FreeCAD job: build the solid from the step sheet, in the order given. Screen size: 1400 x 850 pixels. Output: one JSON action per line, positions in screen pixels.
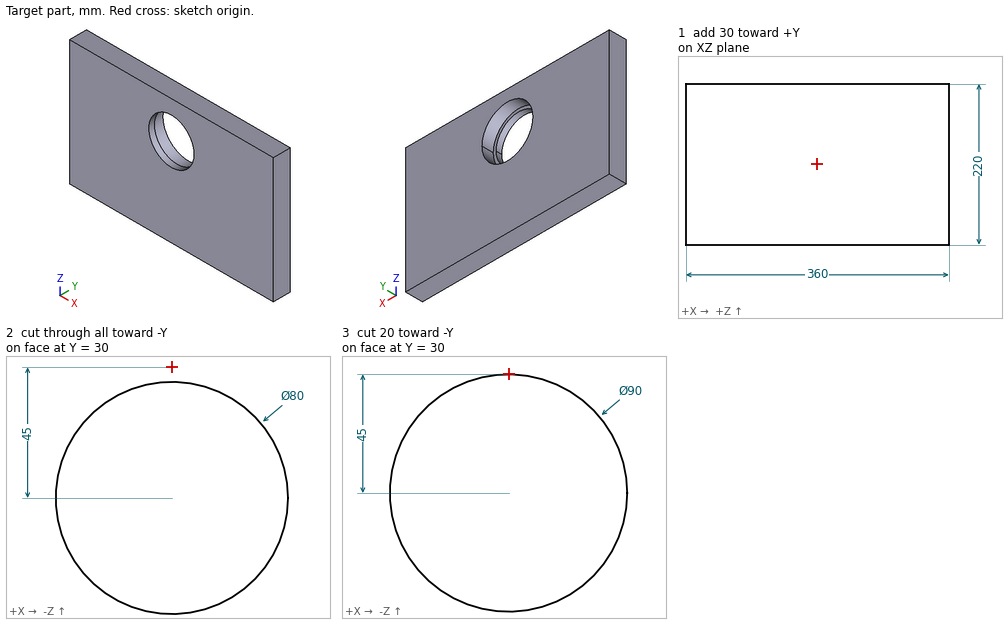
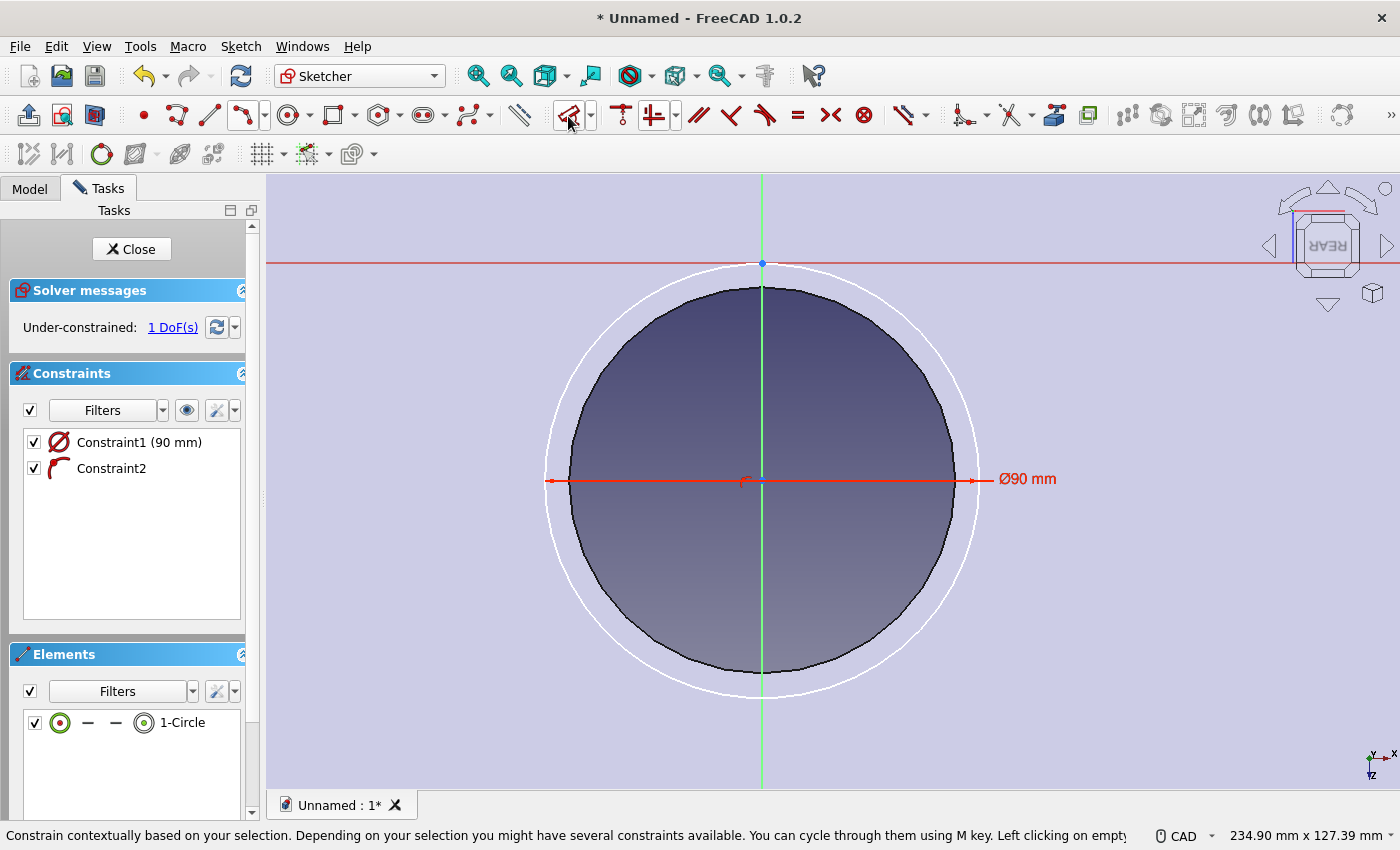
{"action": "left_click", "coordinate": [762, 481]}
{"action": "left_click", "coordinate": [796, 372]}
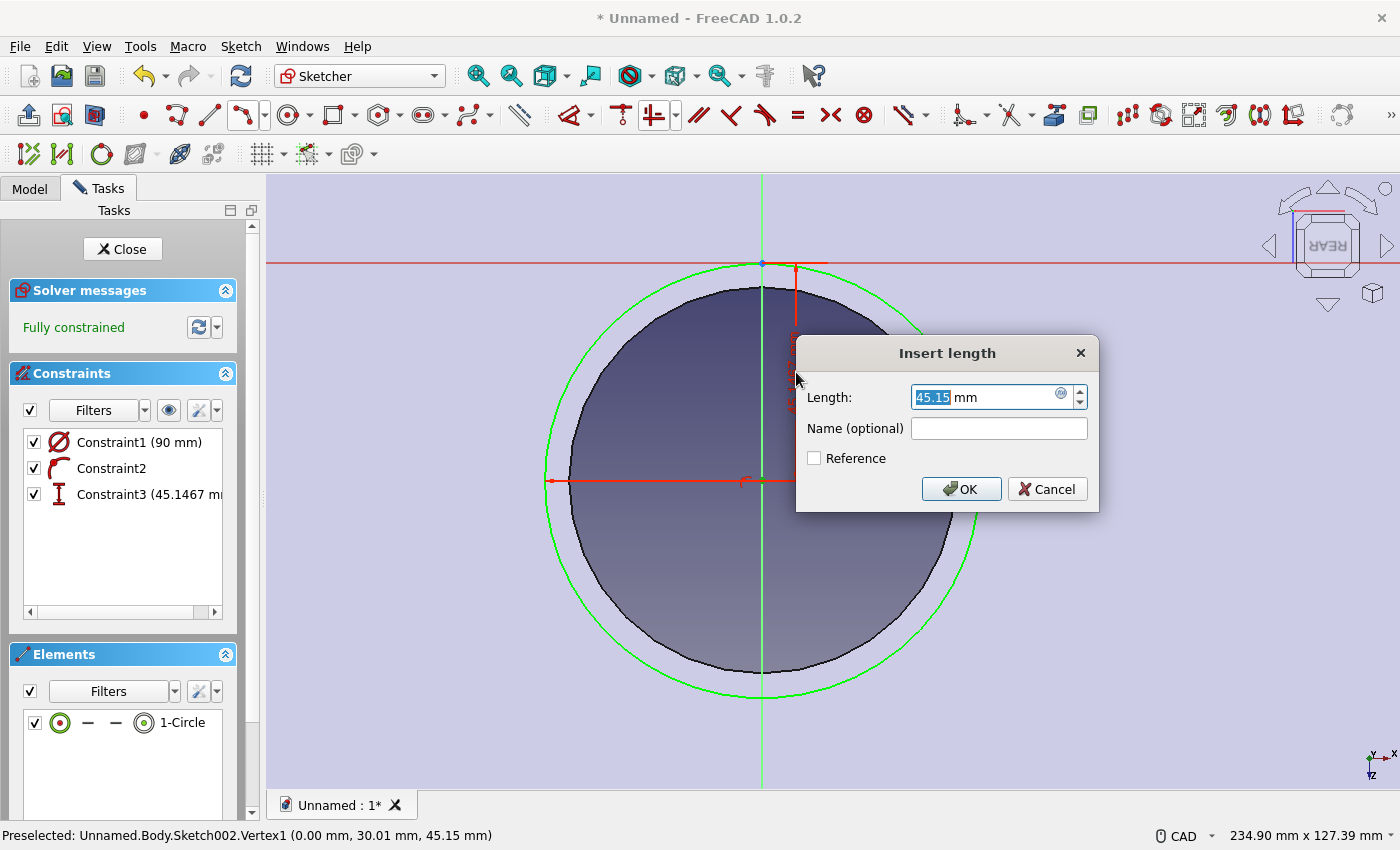
{"action": "type", "text": "45"}
{"action": "key", "text": "Return"}
{"action": "key", "text": "Escape"}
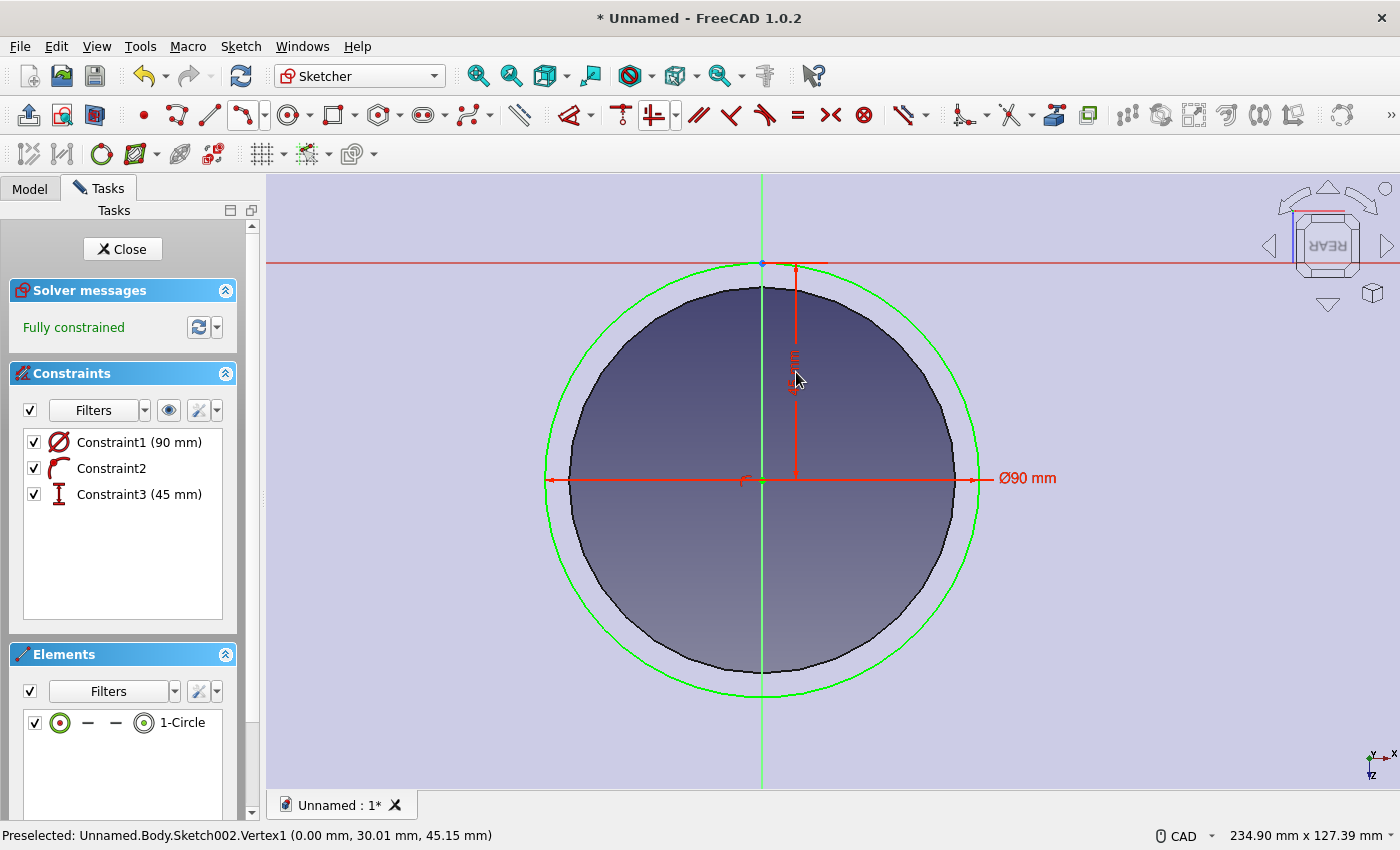
{"action": "left_click", "coordinate": [123, 249]}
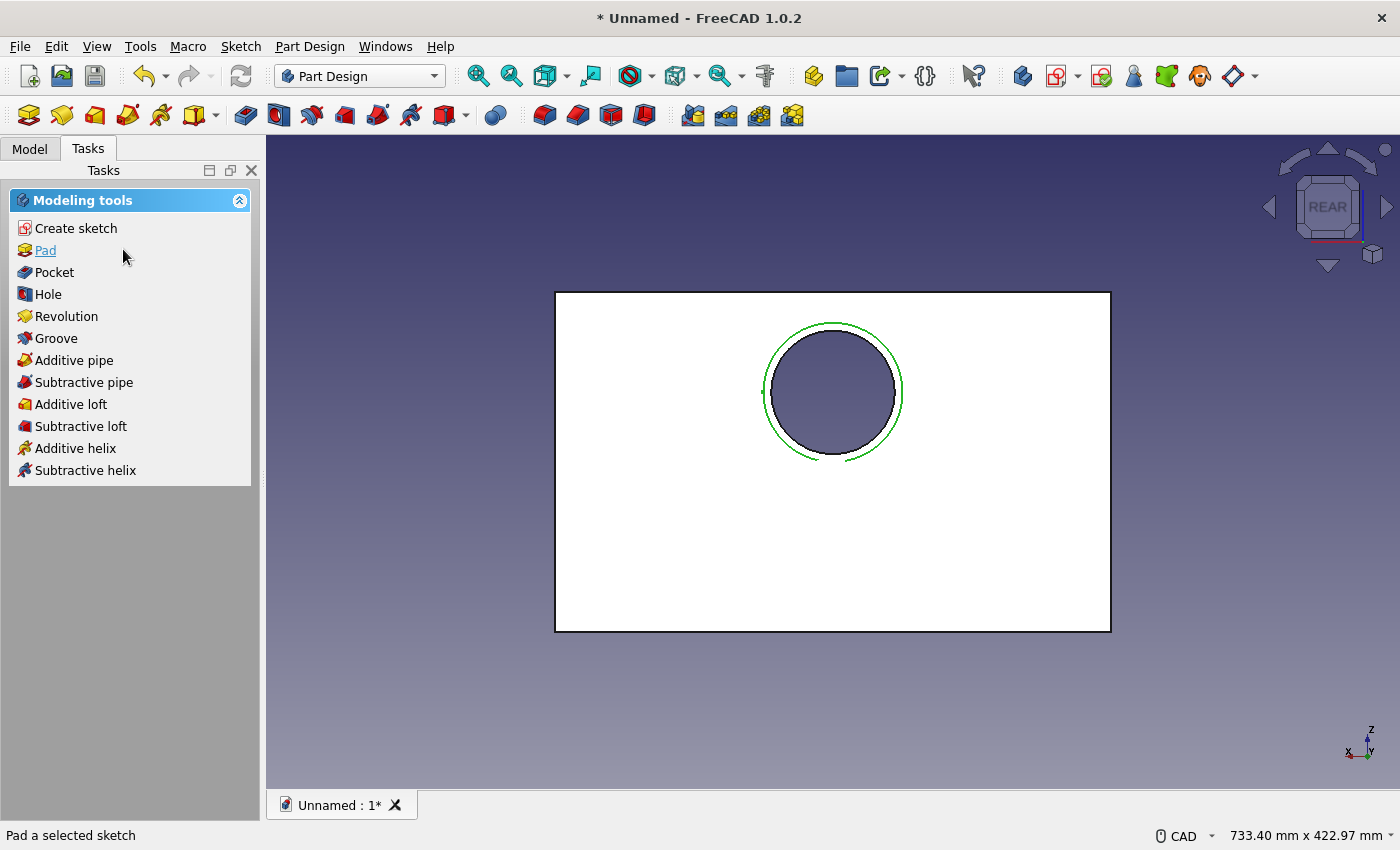
{"action": "left_click", "coordinate": [246, 116]}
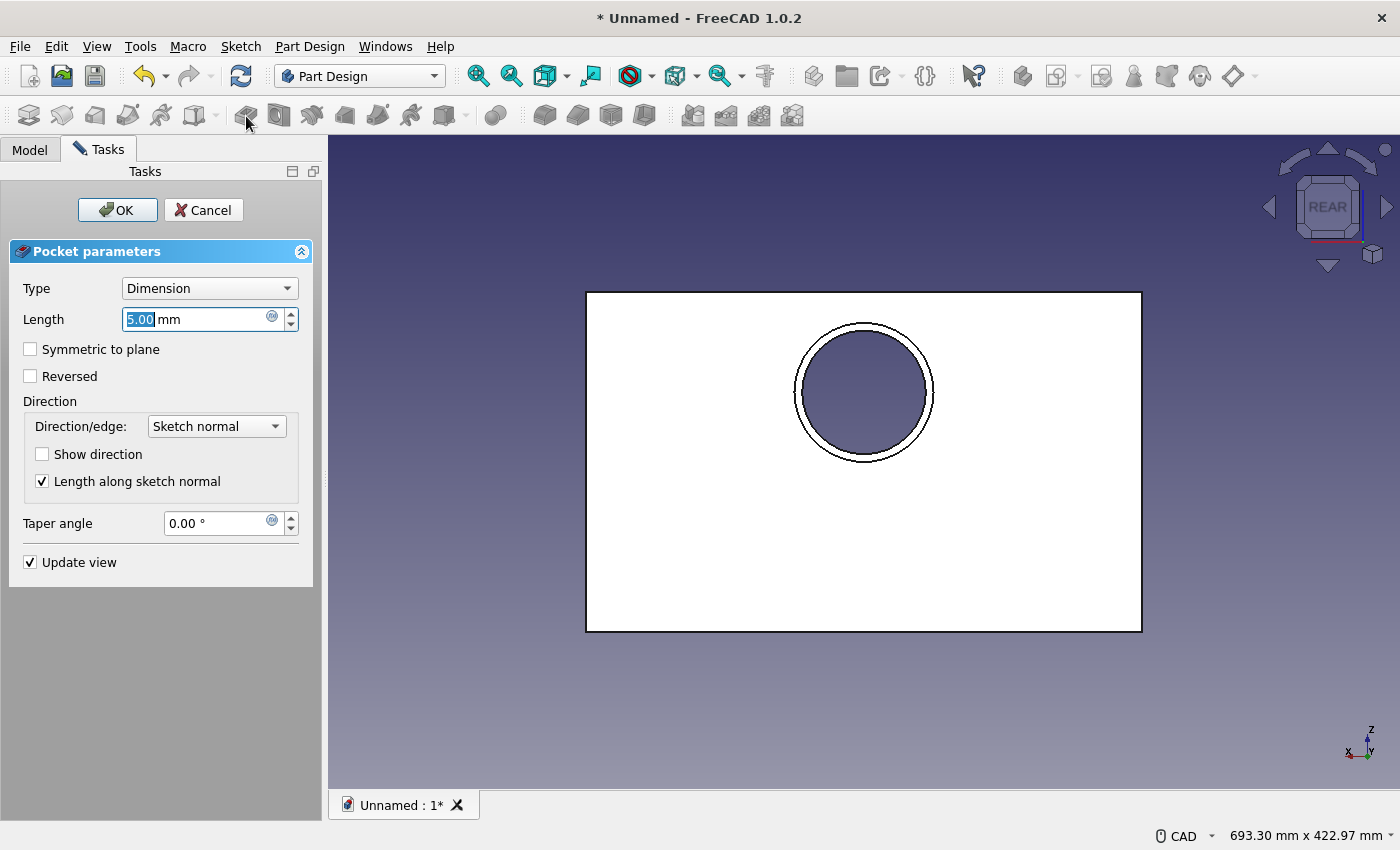
{"action": "type", "text": "20"}
{"action": "key", "text": "Tab"}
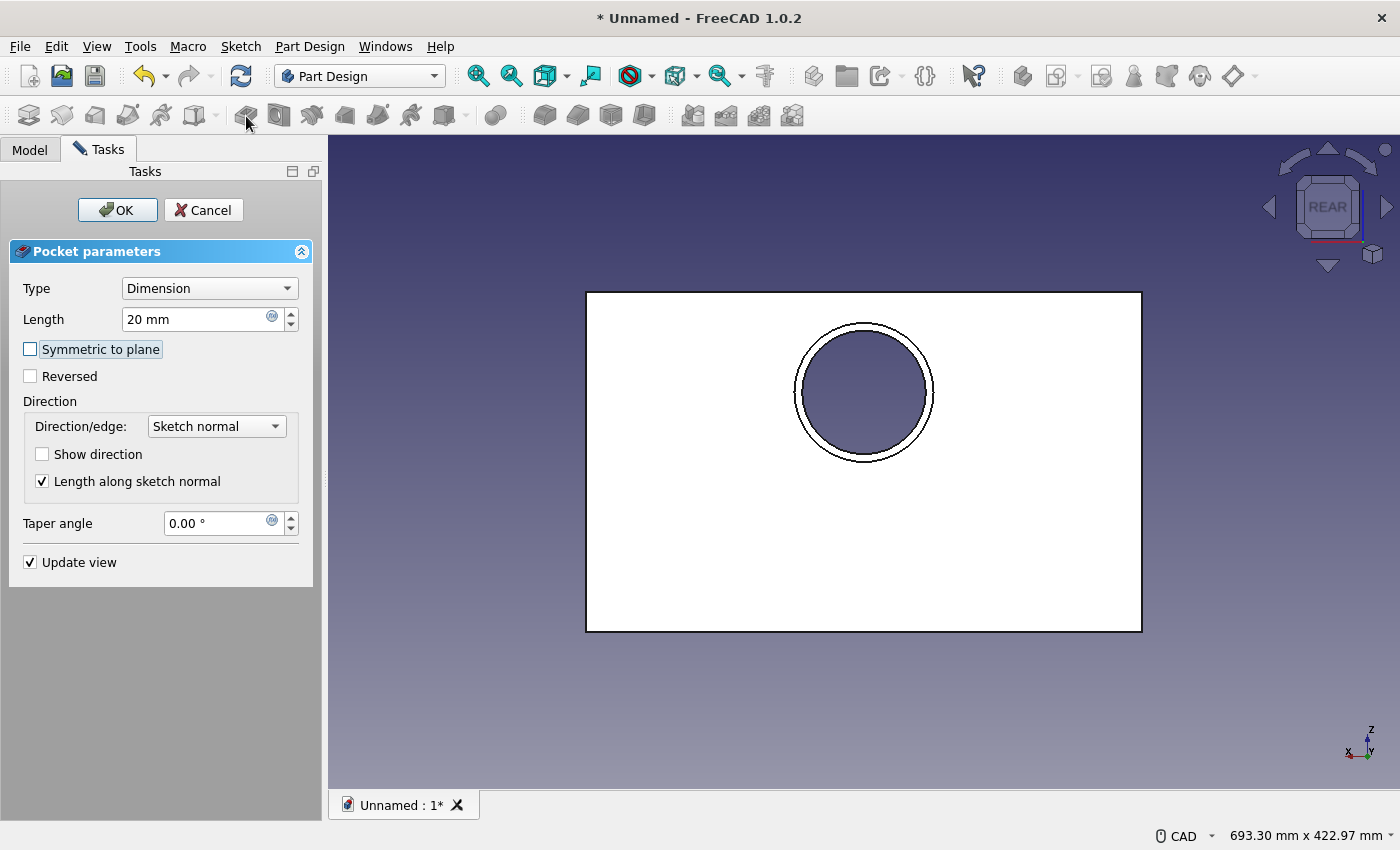
{"action": "left_click", "coordinate": [118, 210]}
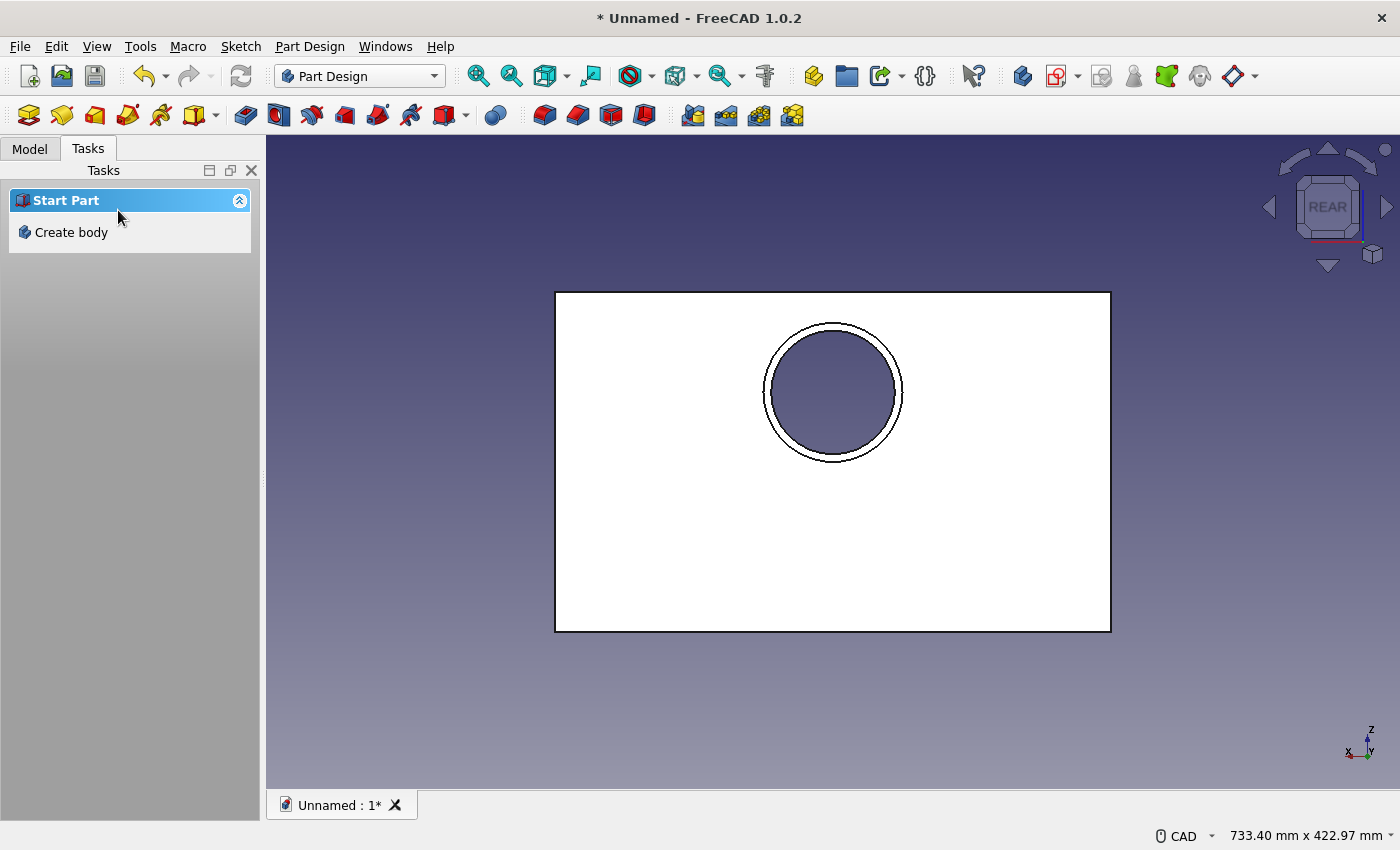
{"action": "key", "text": "0"}